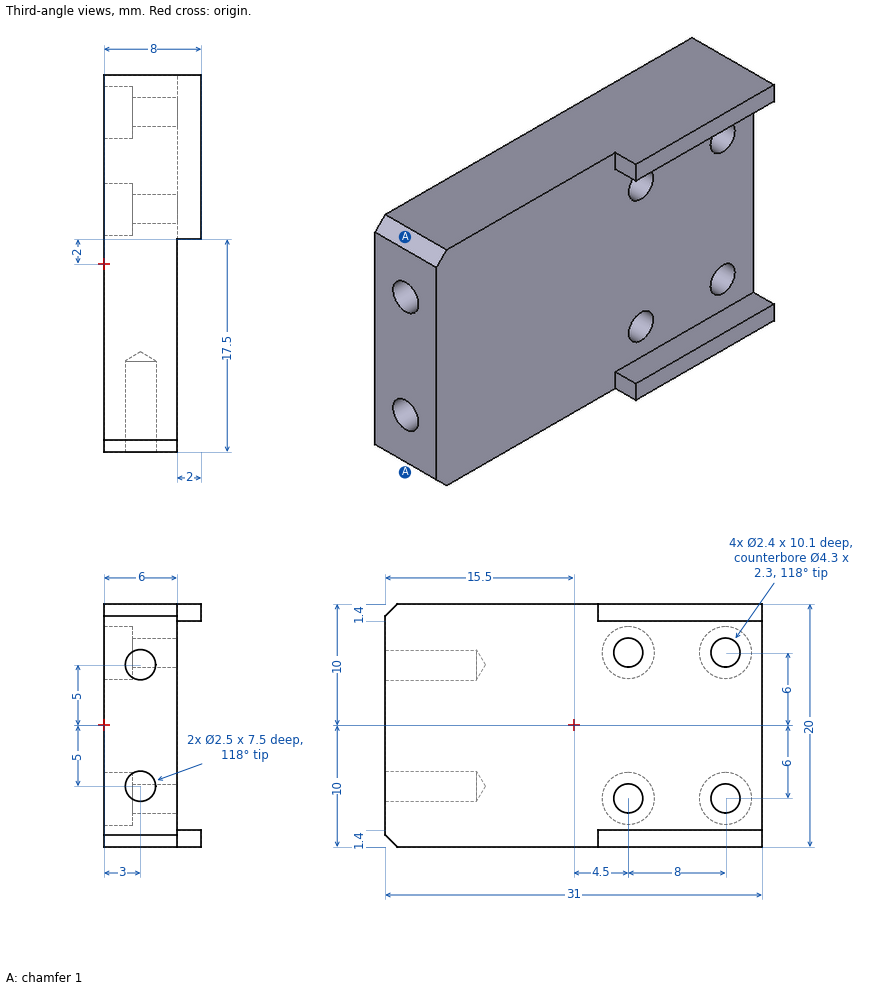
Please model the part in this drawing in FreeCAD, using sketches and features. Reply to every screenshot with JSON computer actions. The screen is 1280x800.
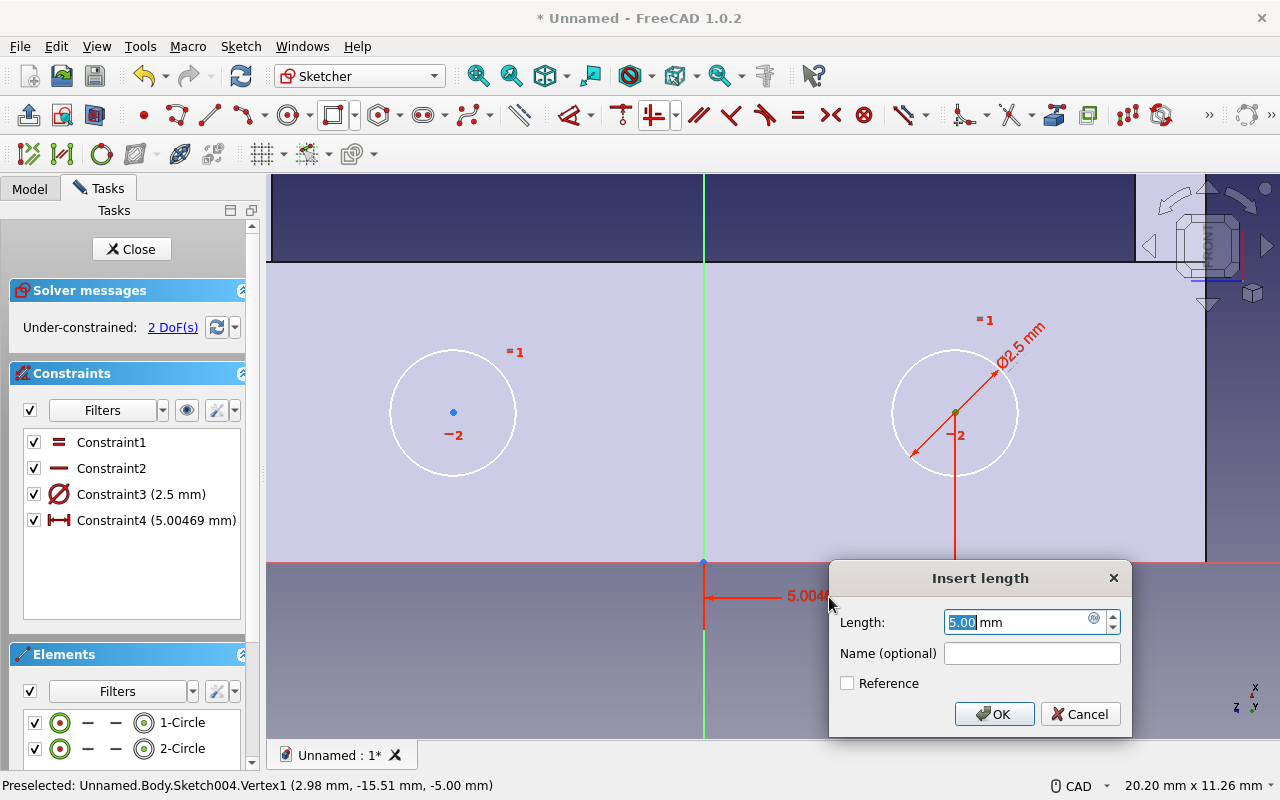
{"action": "type", "text": "5"}
{"action": "key", "text": "Return"}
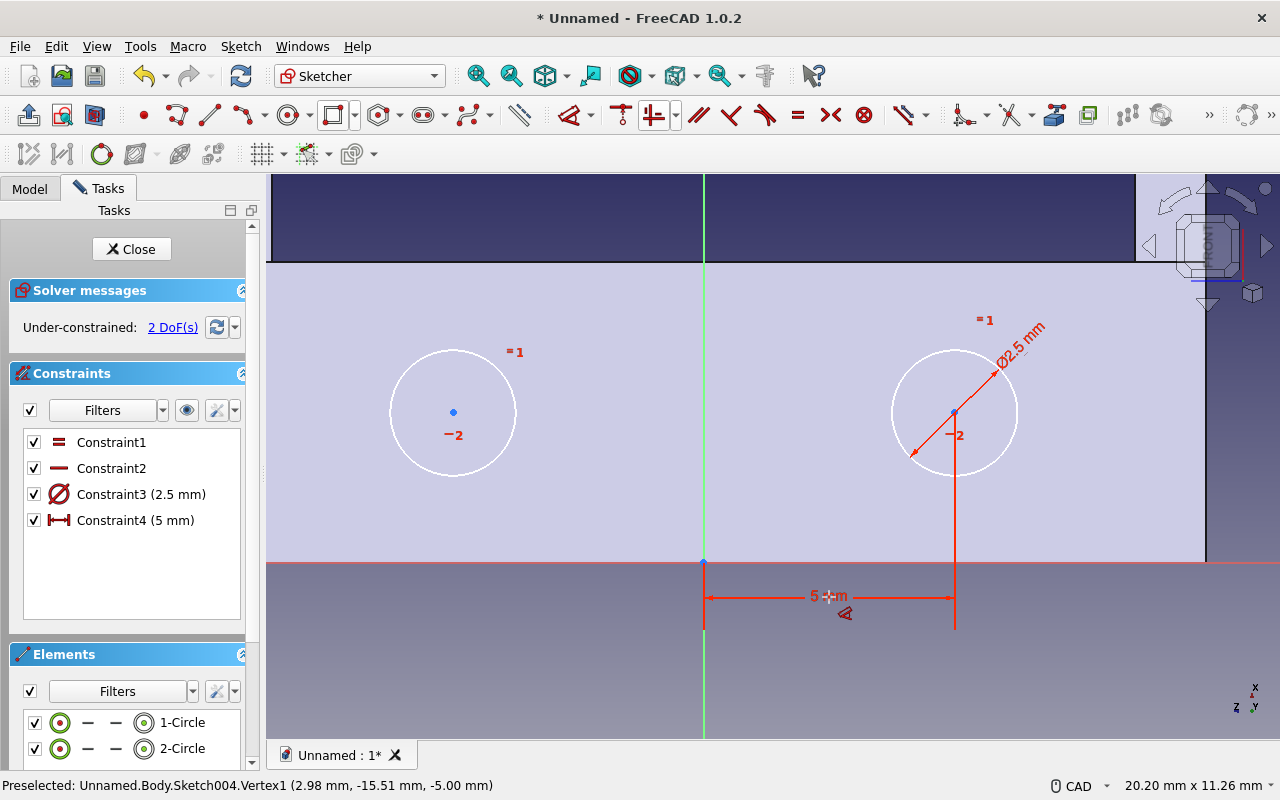
{"action": "left_click", "coordinate": [955, 413]}
{"action": "left_click", "coordinate": [989, 488]}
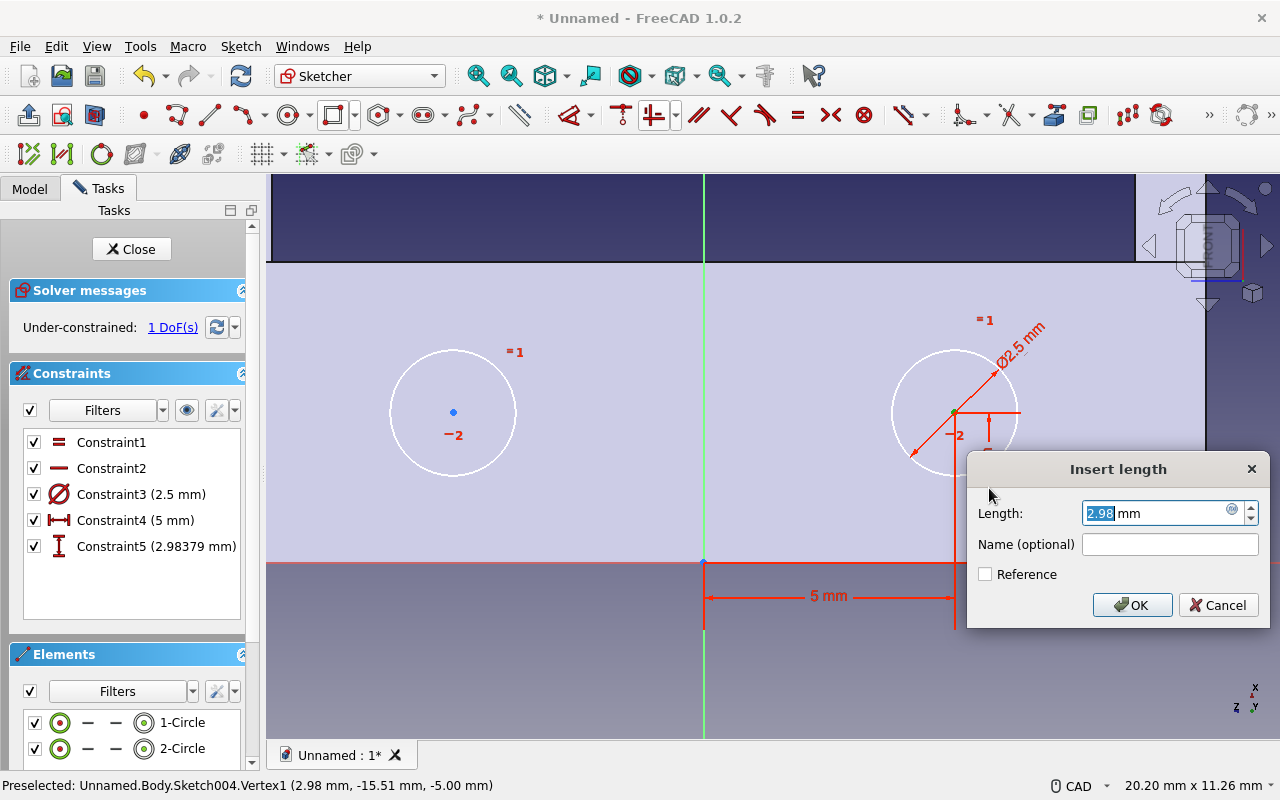
{"action": "type", "text": "3"}
{"action": "key", "text": "Return"}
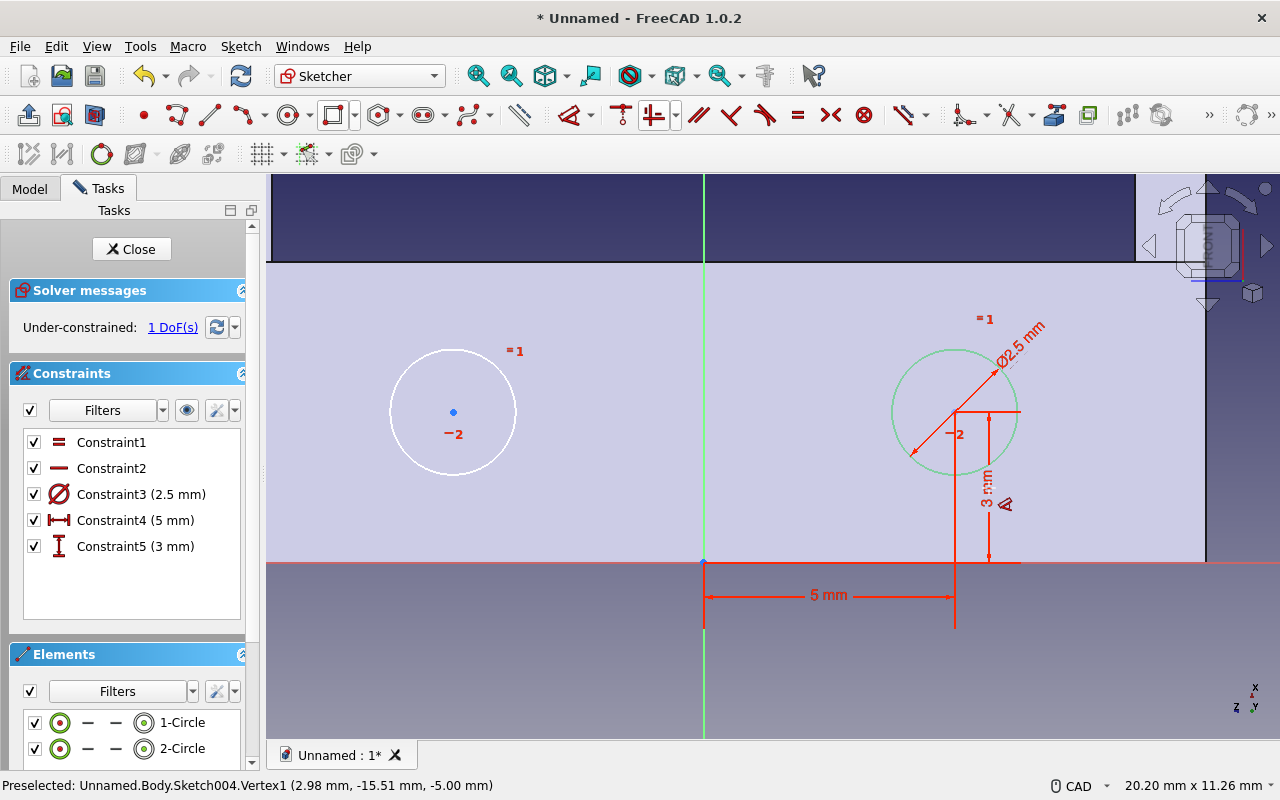
{"action": "left_click", "coordinate": [453, 412]}
{"action": "left_click", "coordinate": [578, 597]}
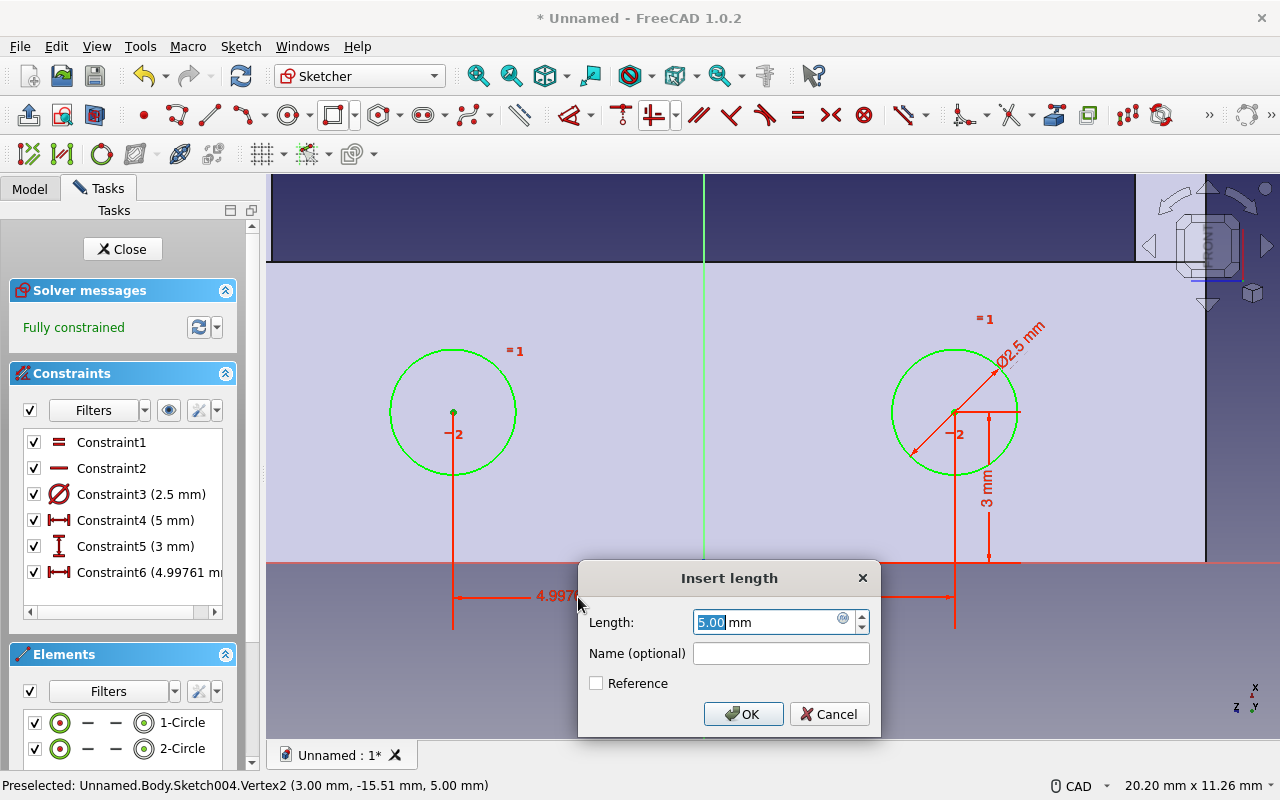
{"action": "type", "text": "5"}
{"action": "key", "text": "Return"}
{"action": "key", "text": "Escape"}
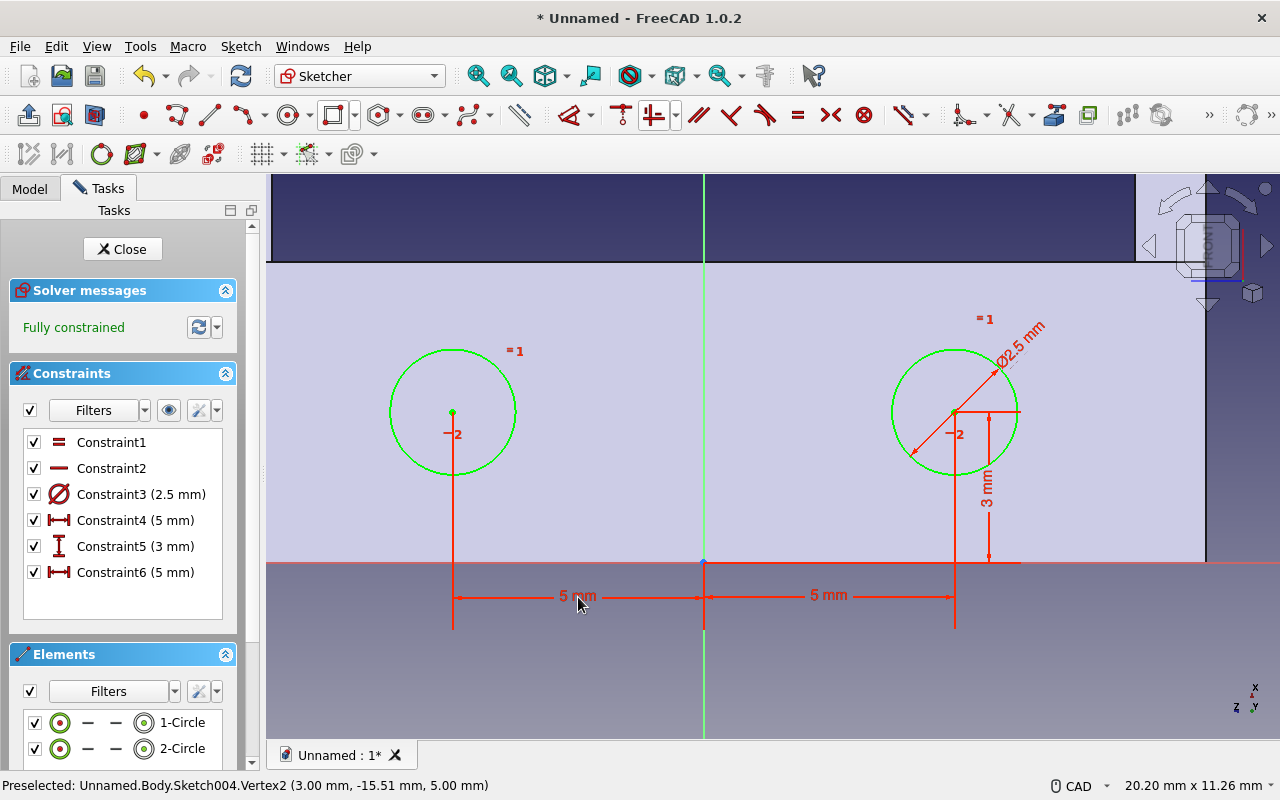
{"action": "left_click", "coordinate": [123, 249]}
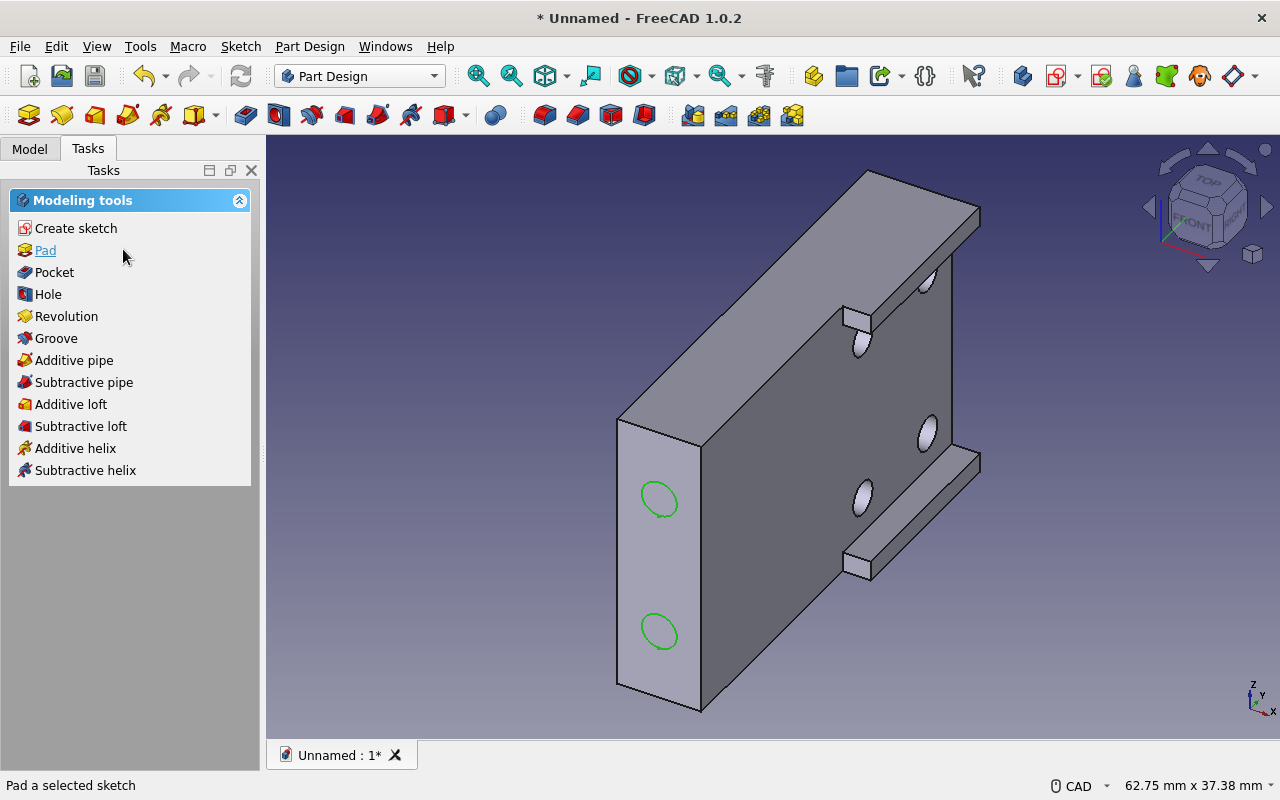
{"action": "left_click", "coordinate": [279, 116]}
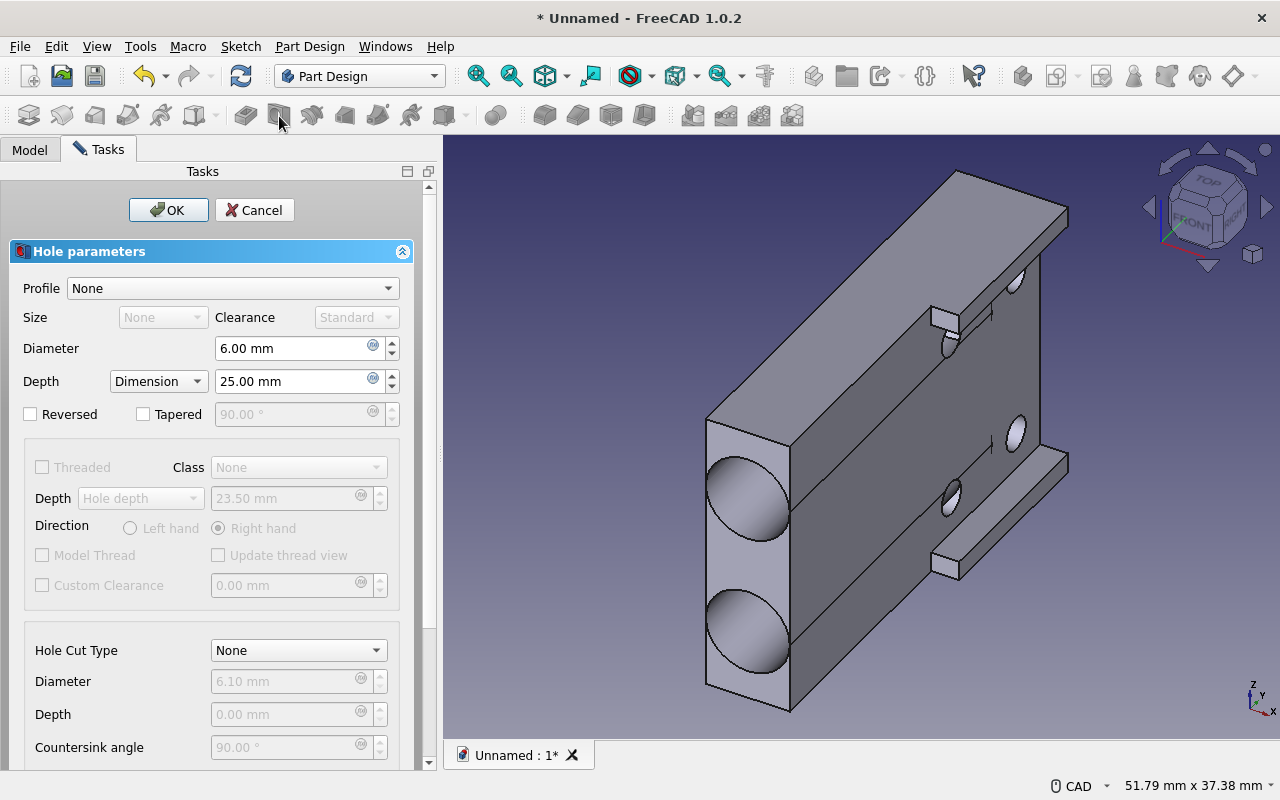
{"action": "triple_click", "coordinate": [300, 348]}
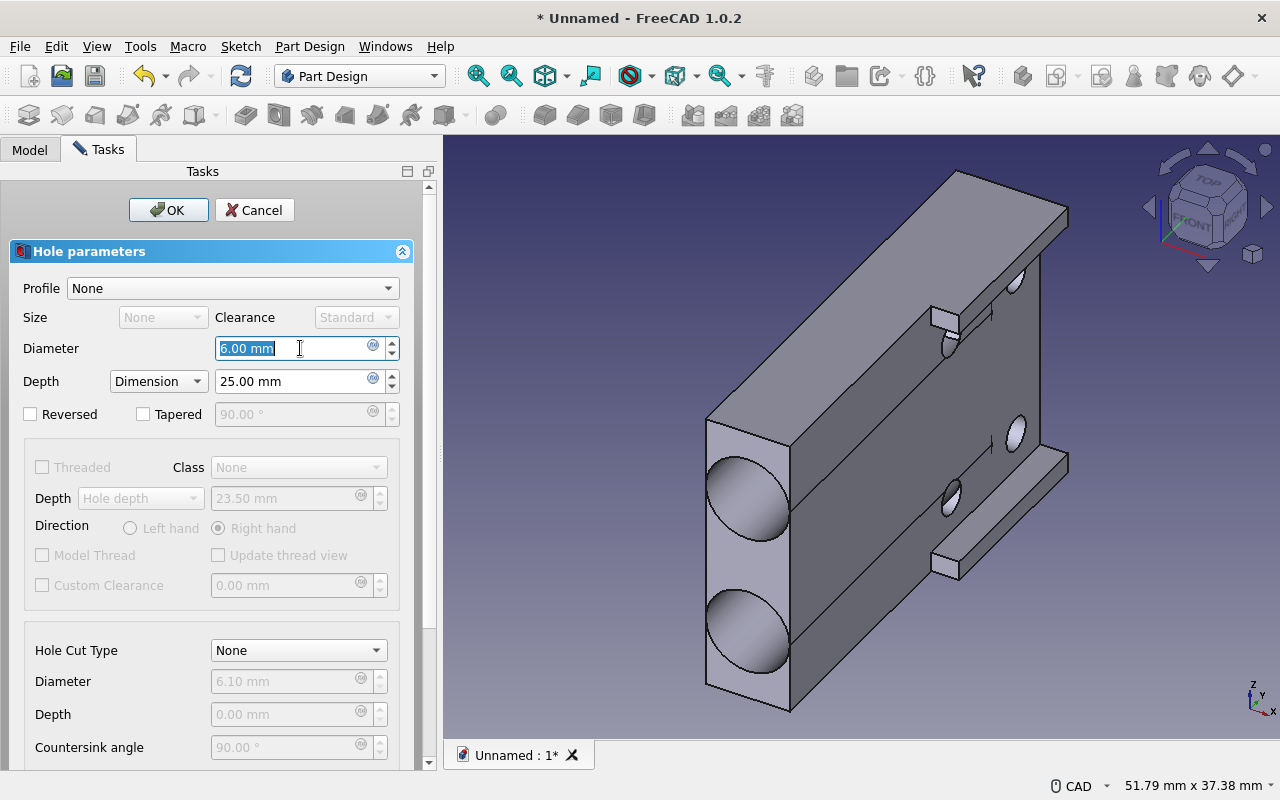
{"action": "type", "text": "2.5"}
{"action": "key", "text": "Tab"}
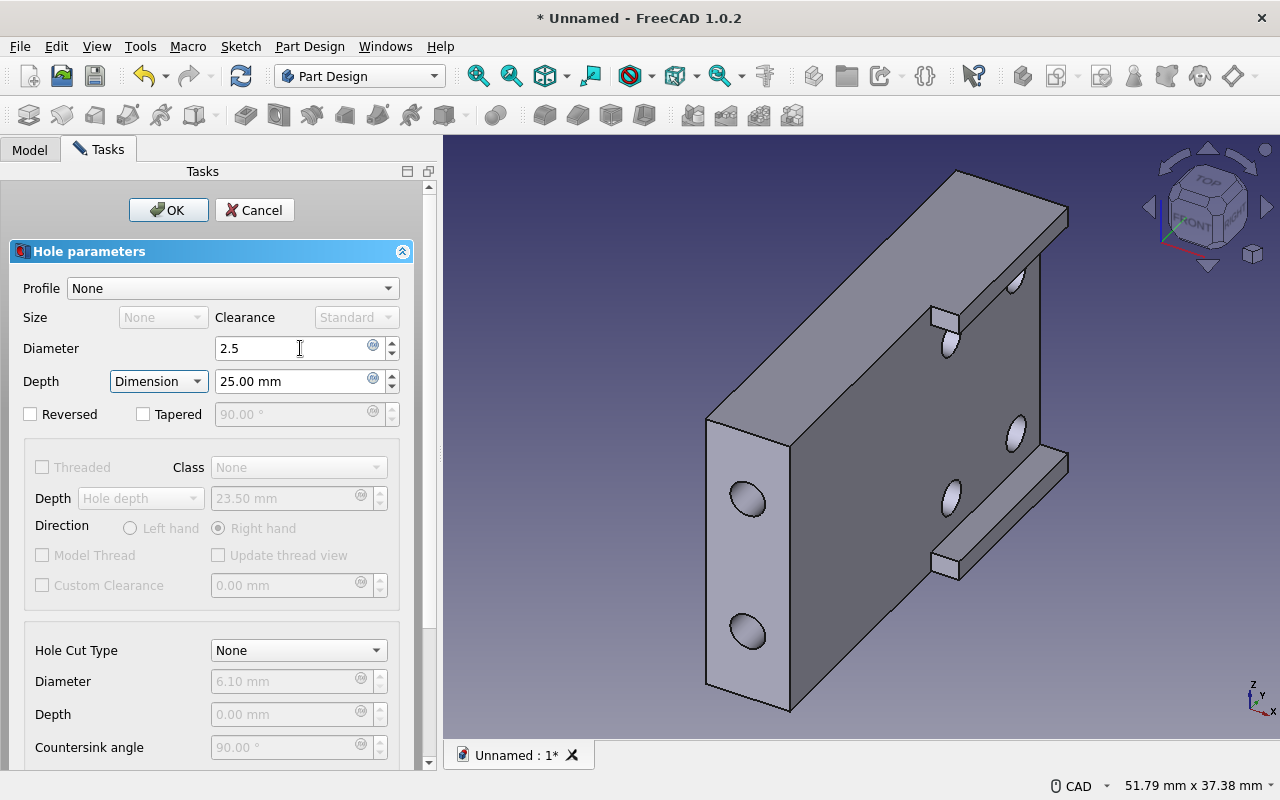
{"action": "triple_click", "coordinate": [300, 382]}